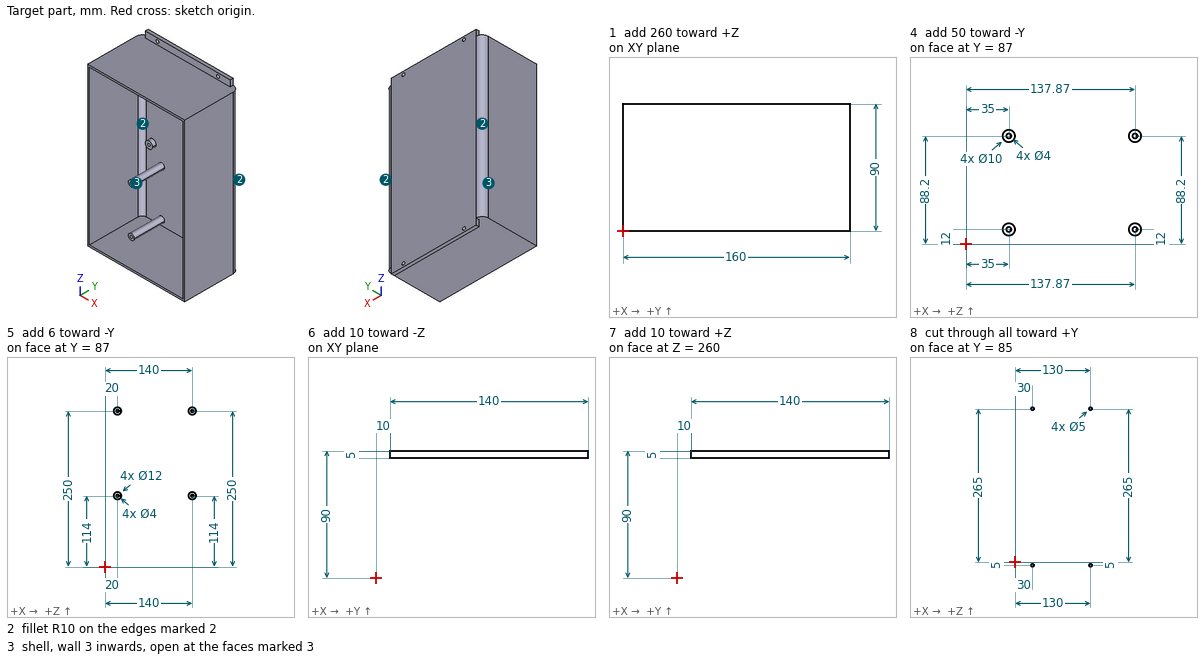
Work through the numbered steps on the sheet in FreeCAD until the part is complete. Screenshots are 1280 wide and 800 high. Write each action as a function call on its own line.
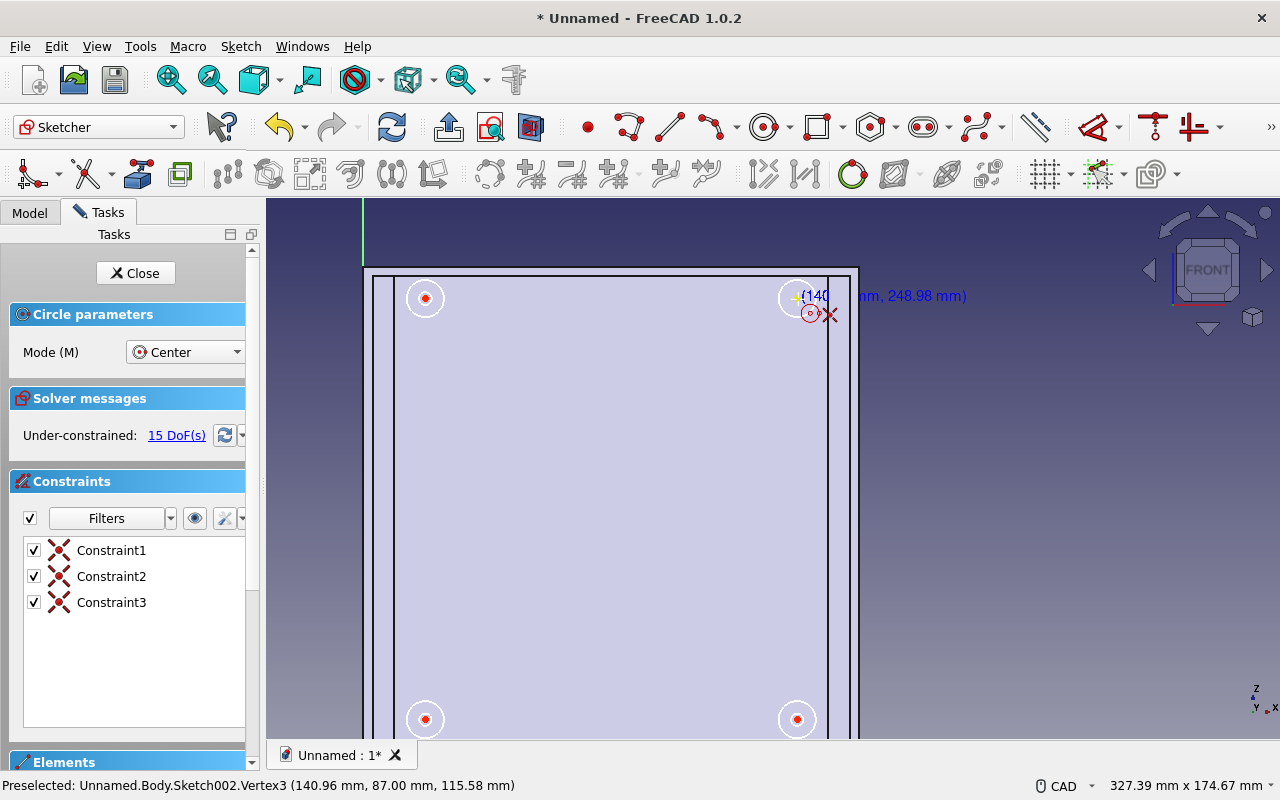
click(797, 299)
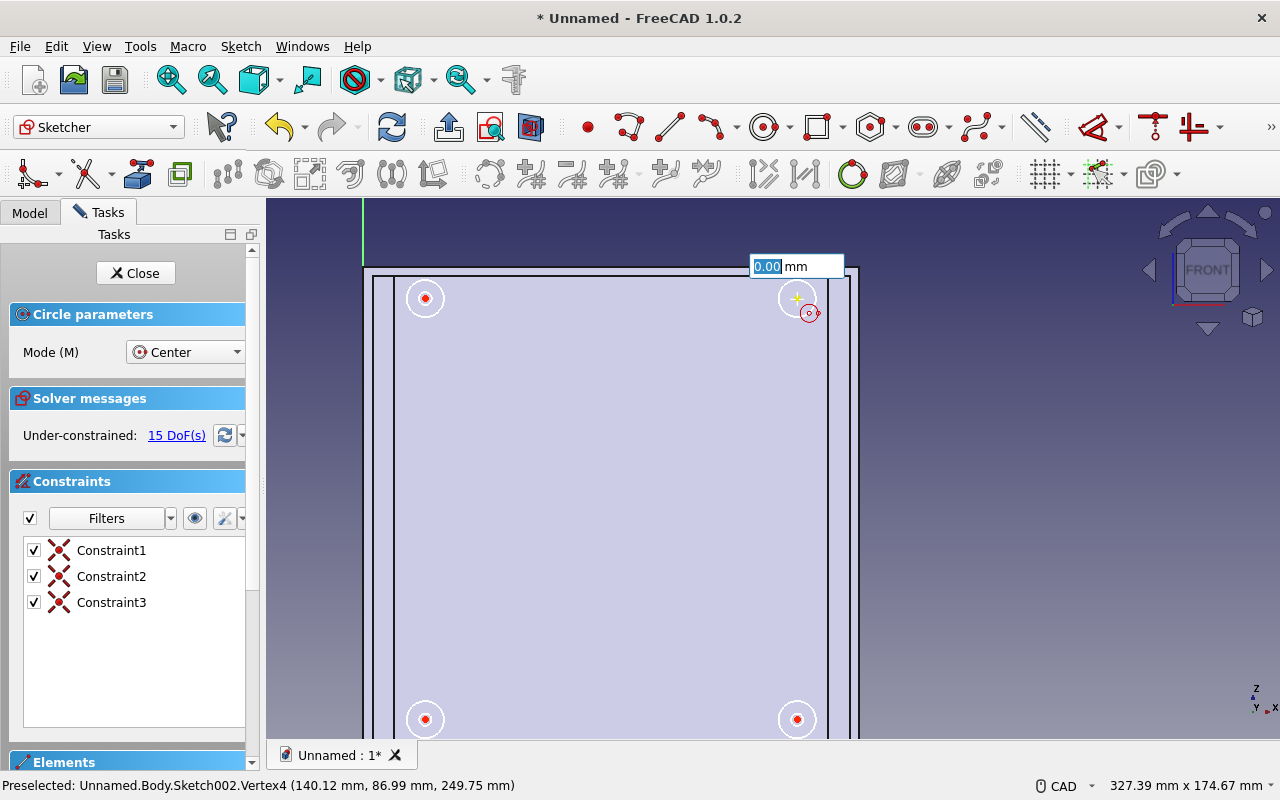
scroll(801, 293, up, 5)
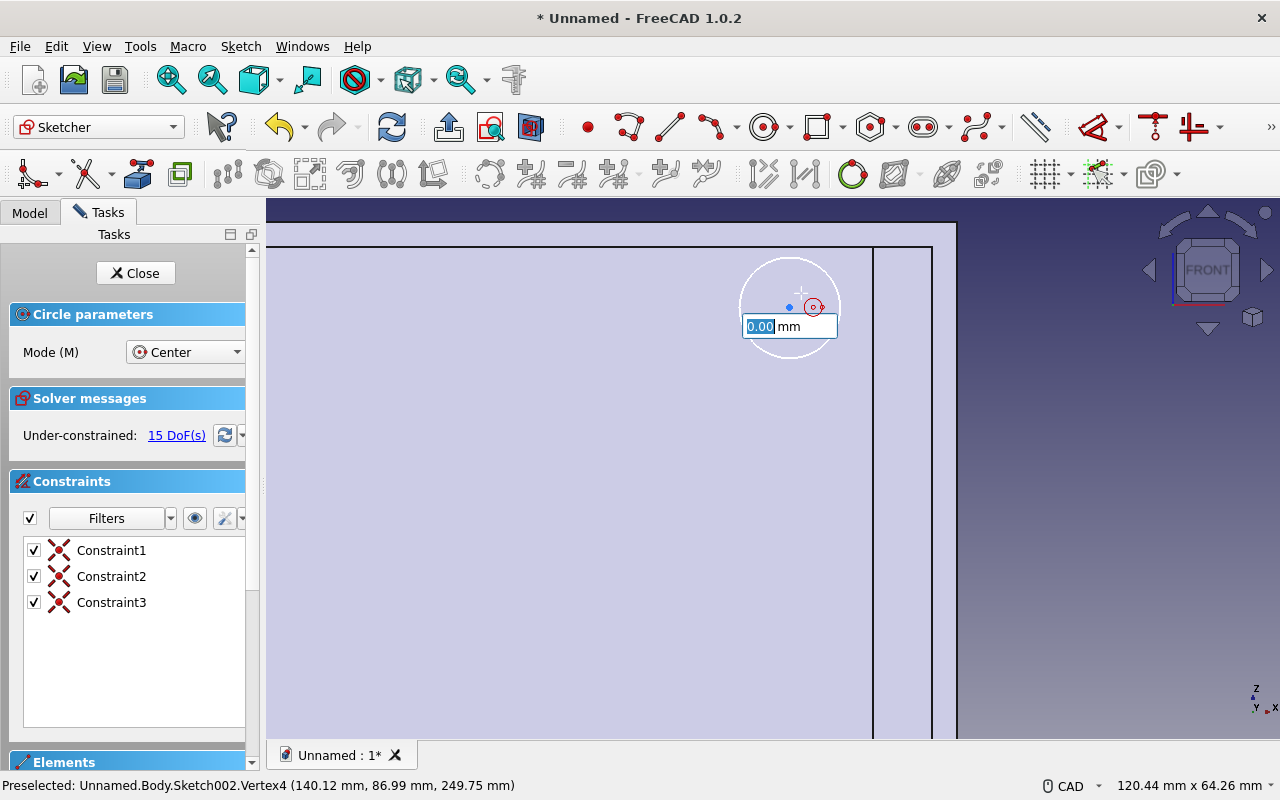
click(801, 294)
key(Escape)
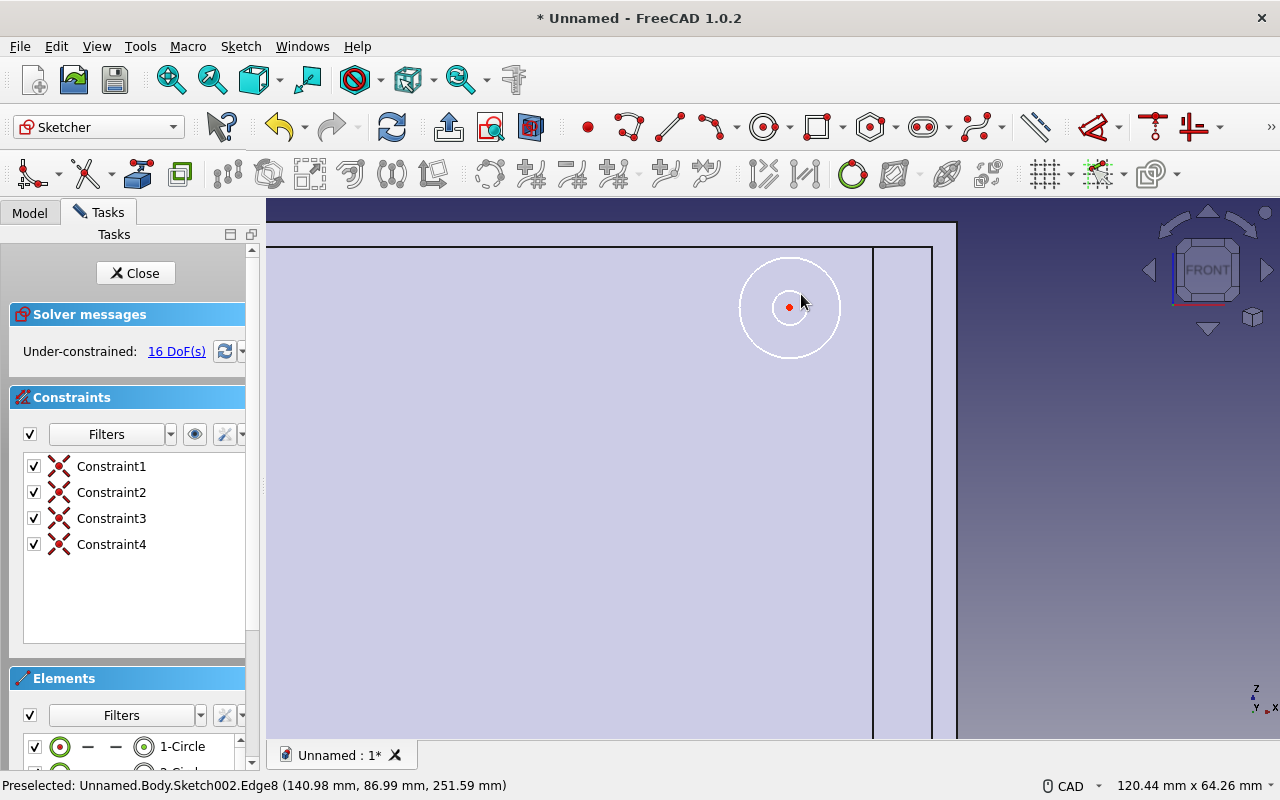
scroll(799, 297, down, 9)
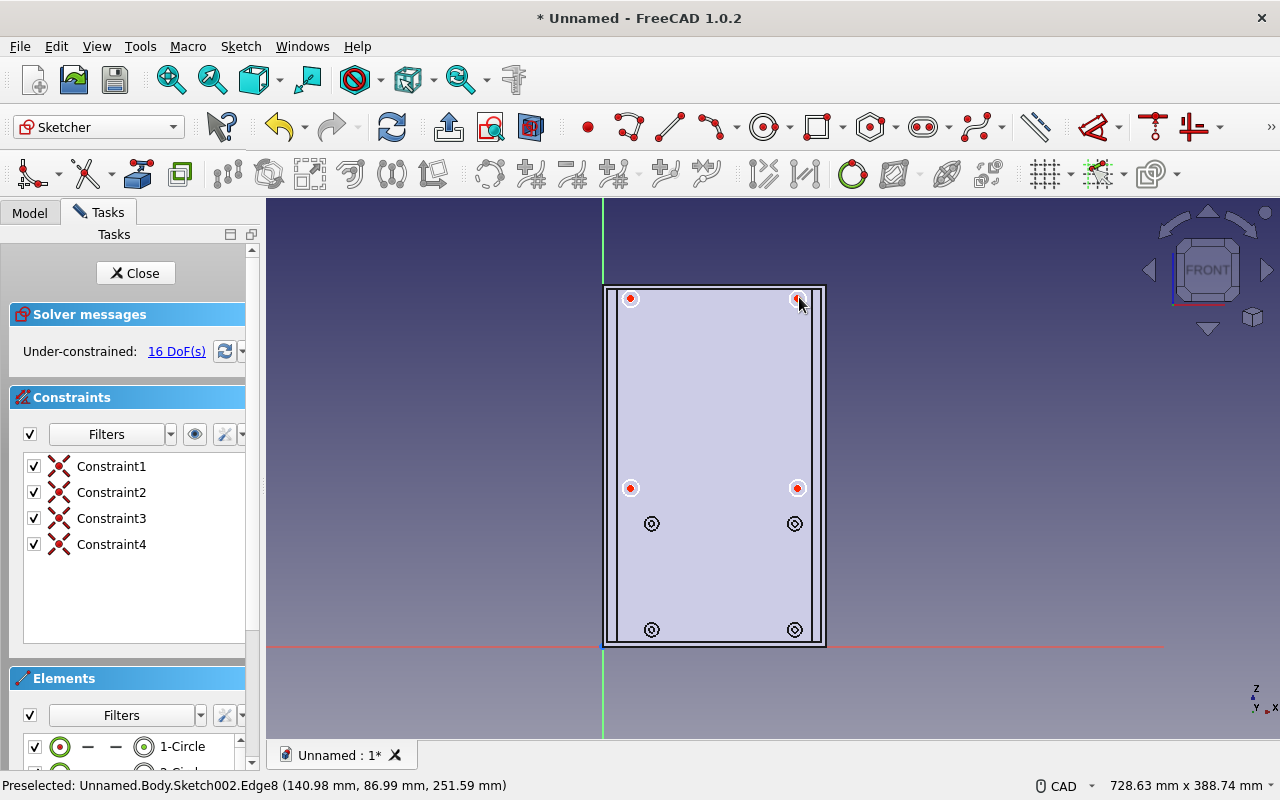
scroll(637, 482, up, 5)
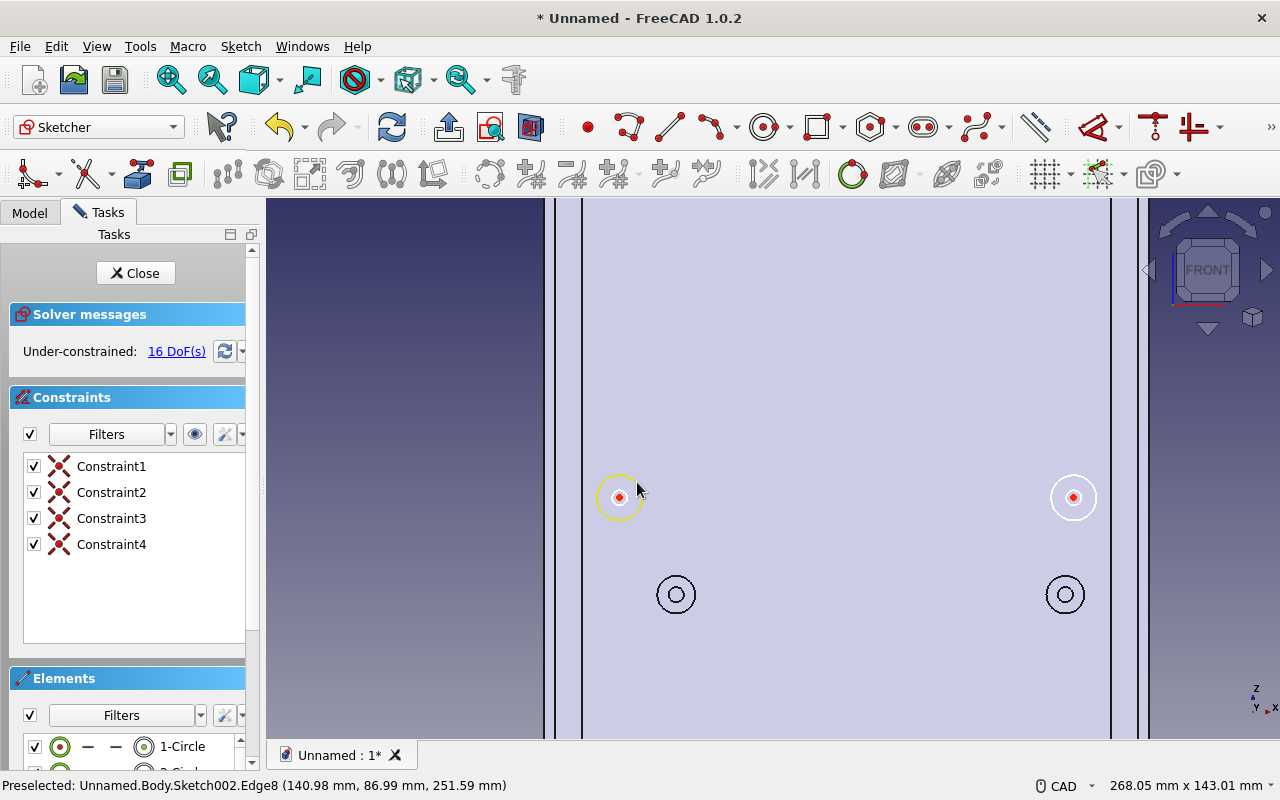
click(636, 482)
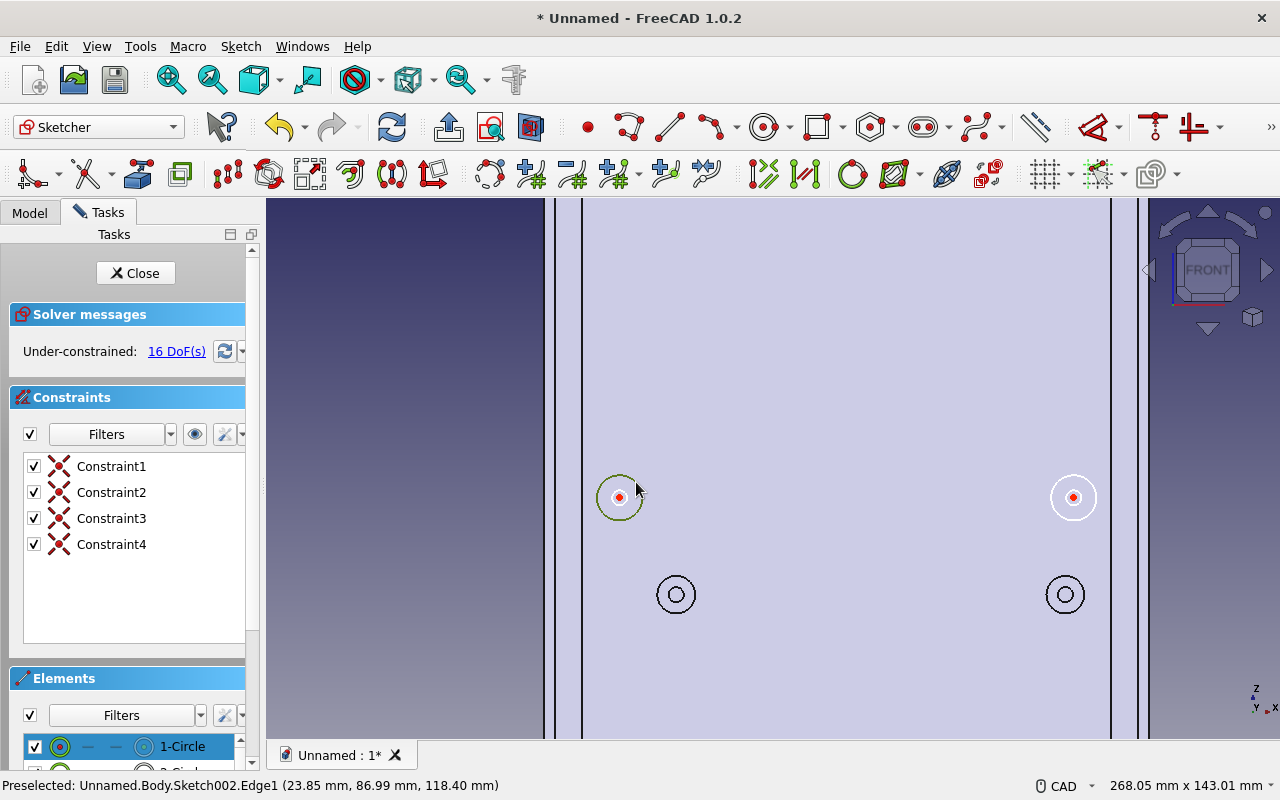
scroll(637, 483, down, 5)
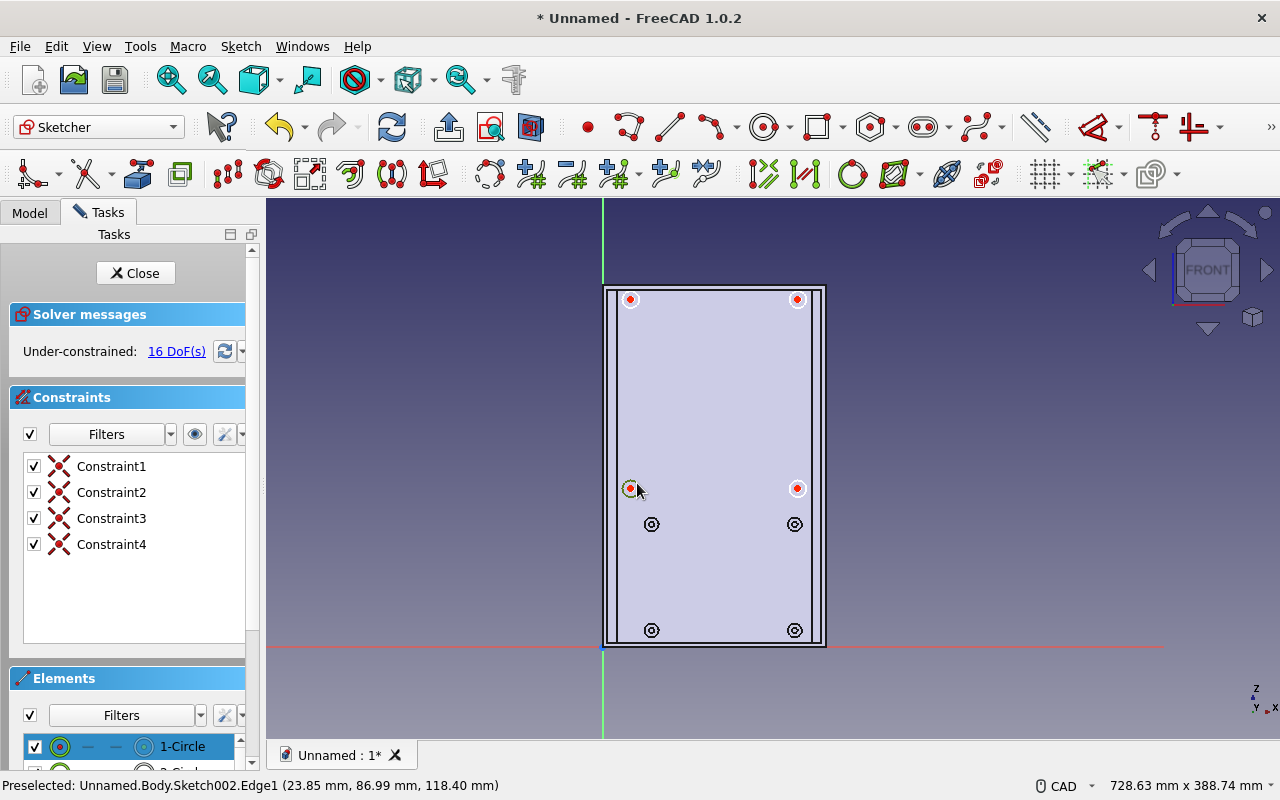
scroll(637, 294, up, 5)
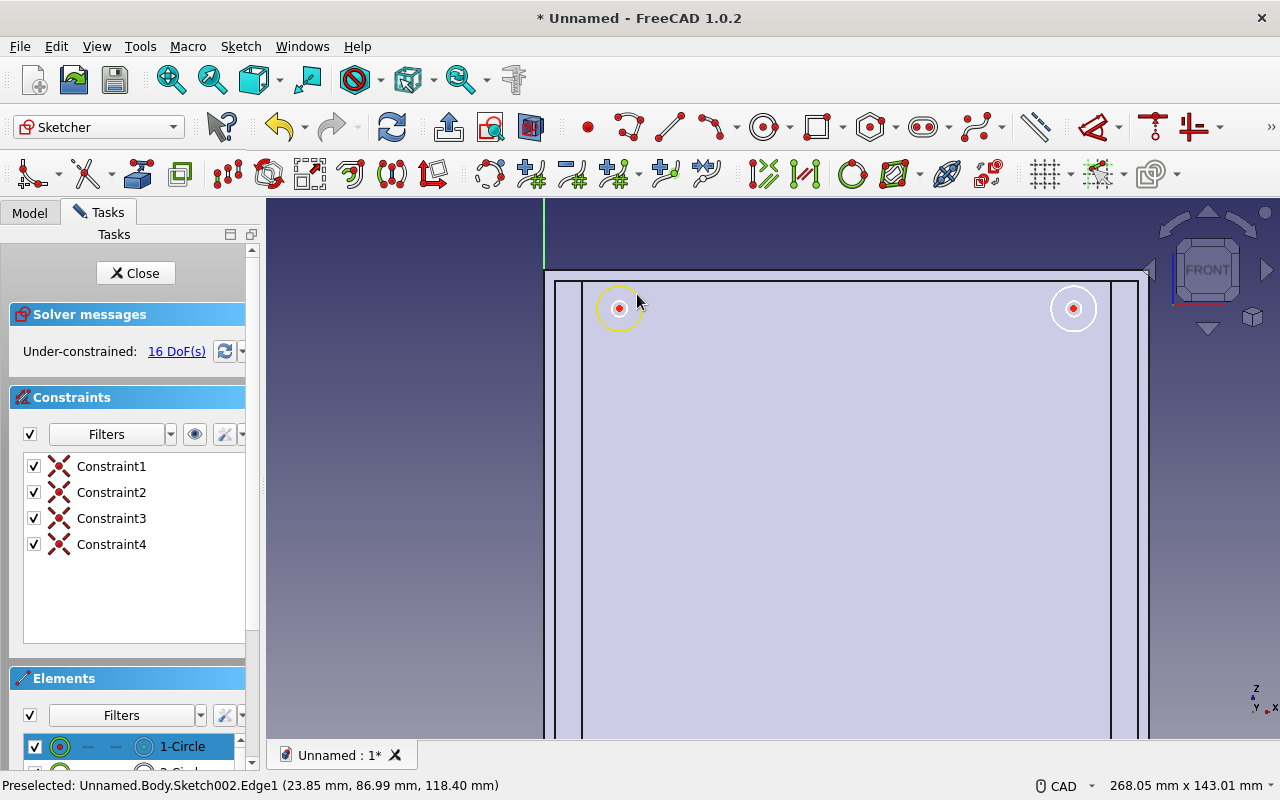
click(636, 293)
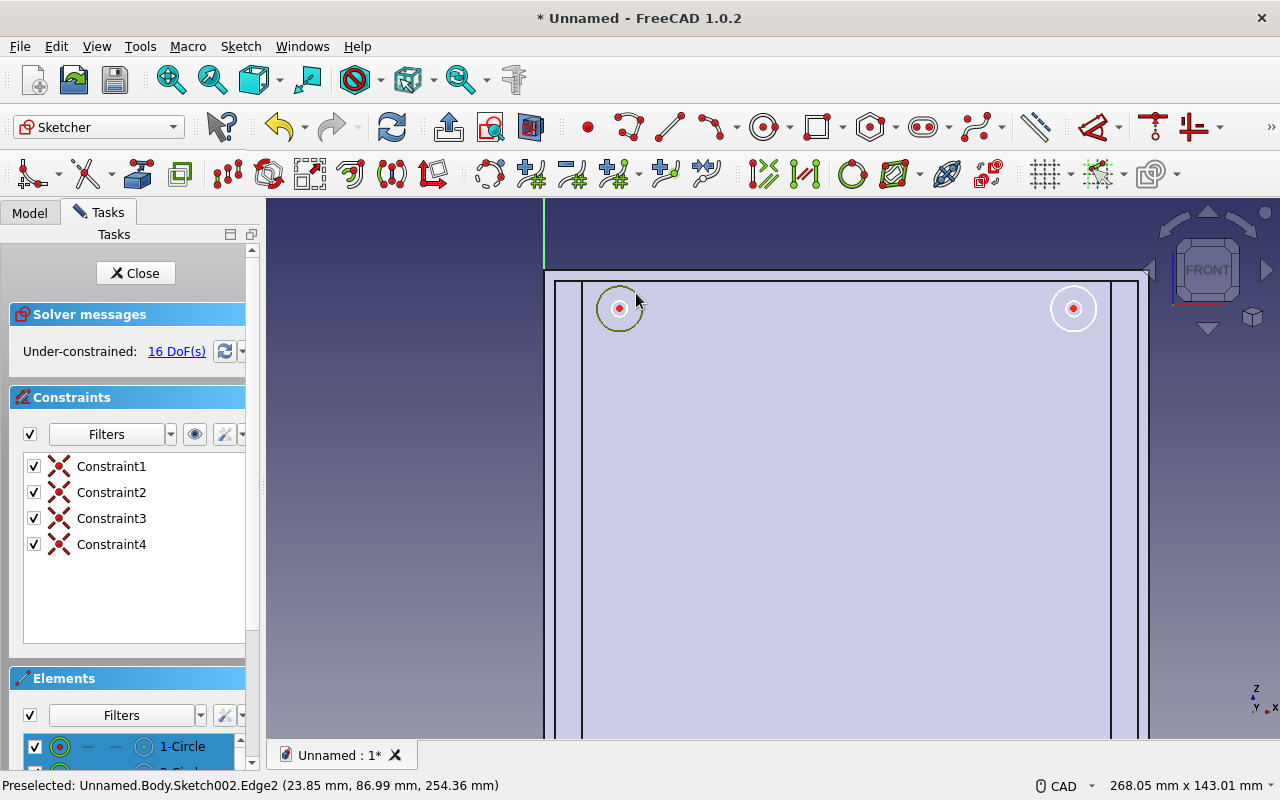
scroll(637, 293, down, 5)